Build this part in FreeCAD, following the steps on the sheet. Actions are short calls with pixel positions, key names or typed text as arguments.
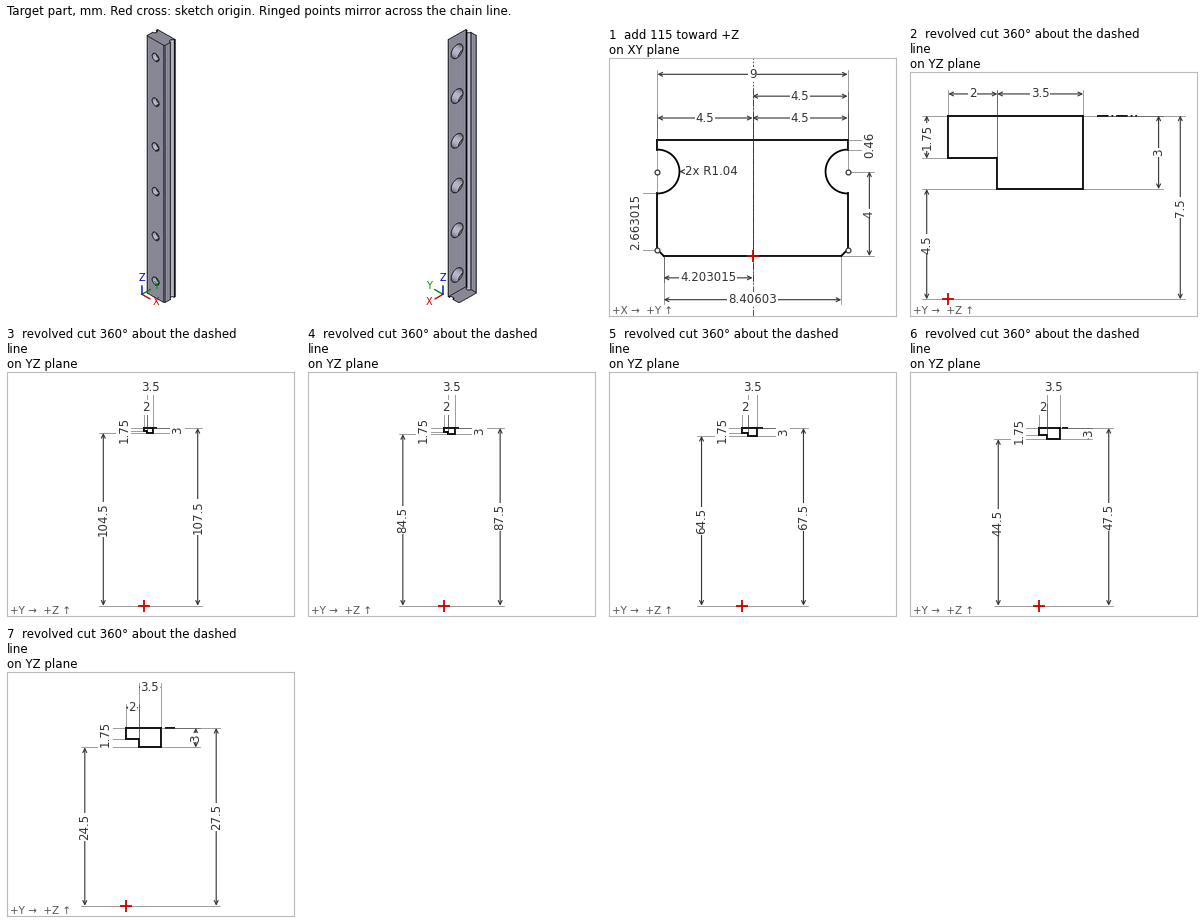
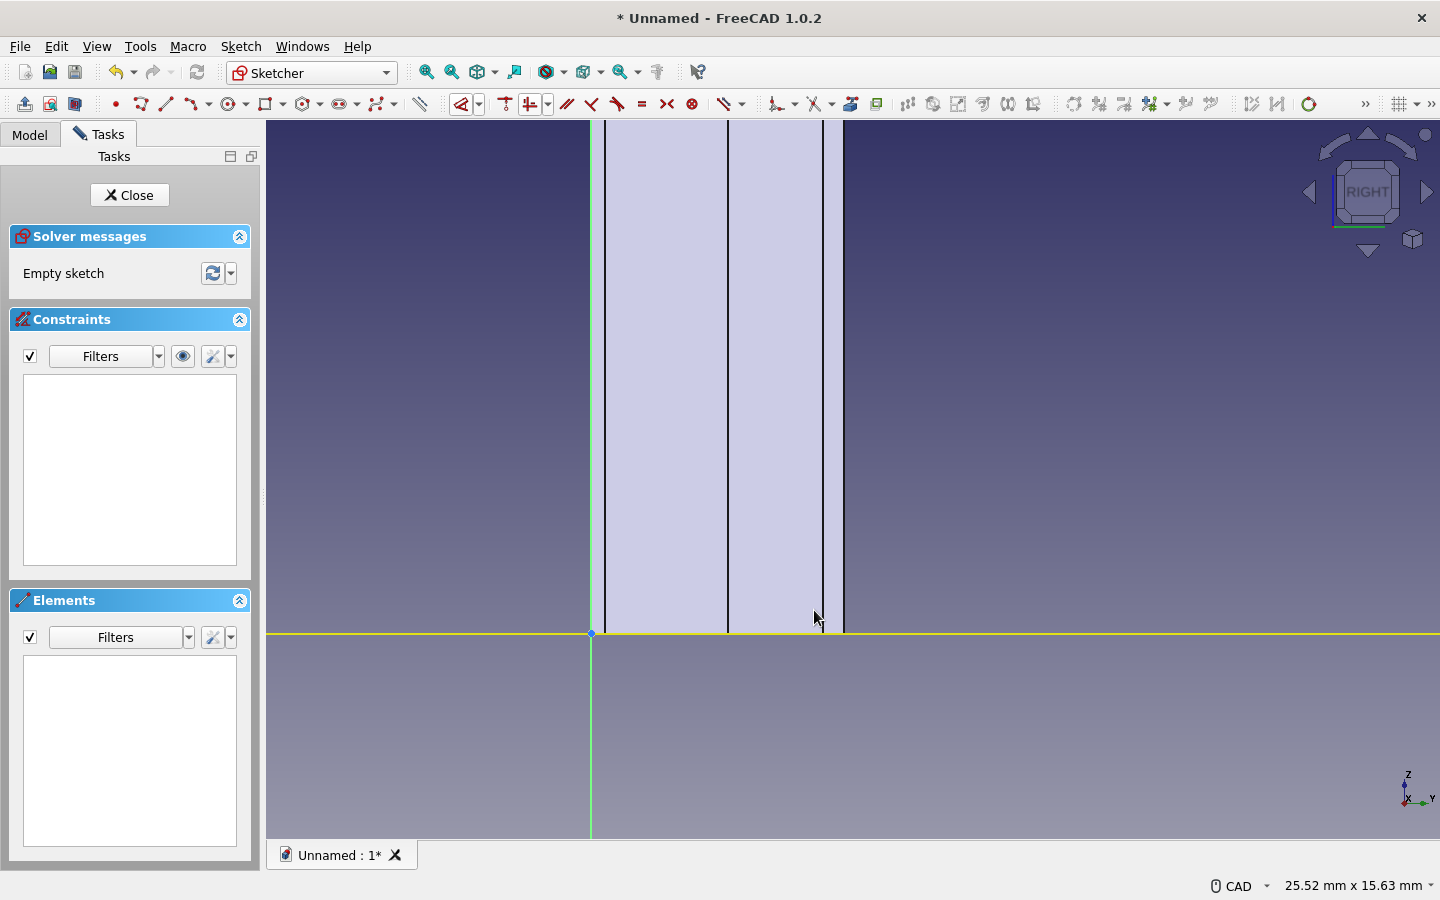
scroll(736, 424, up, 2)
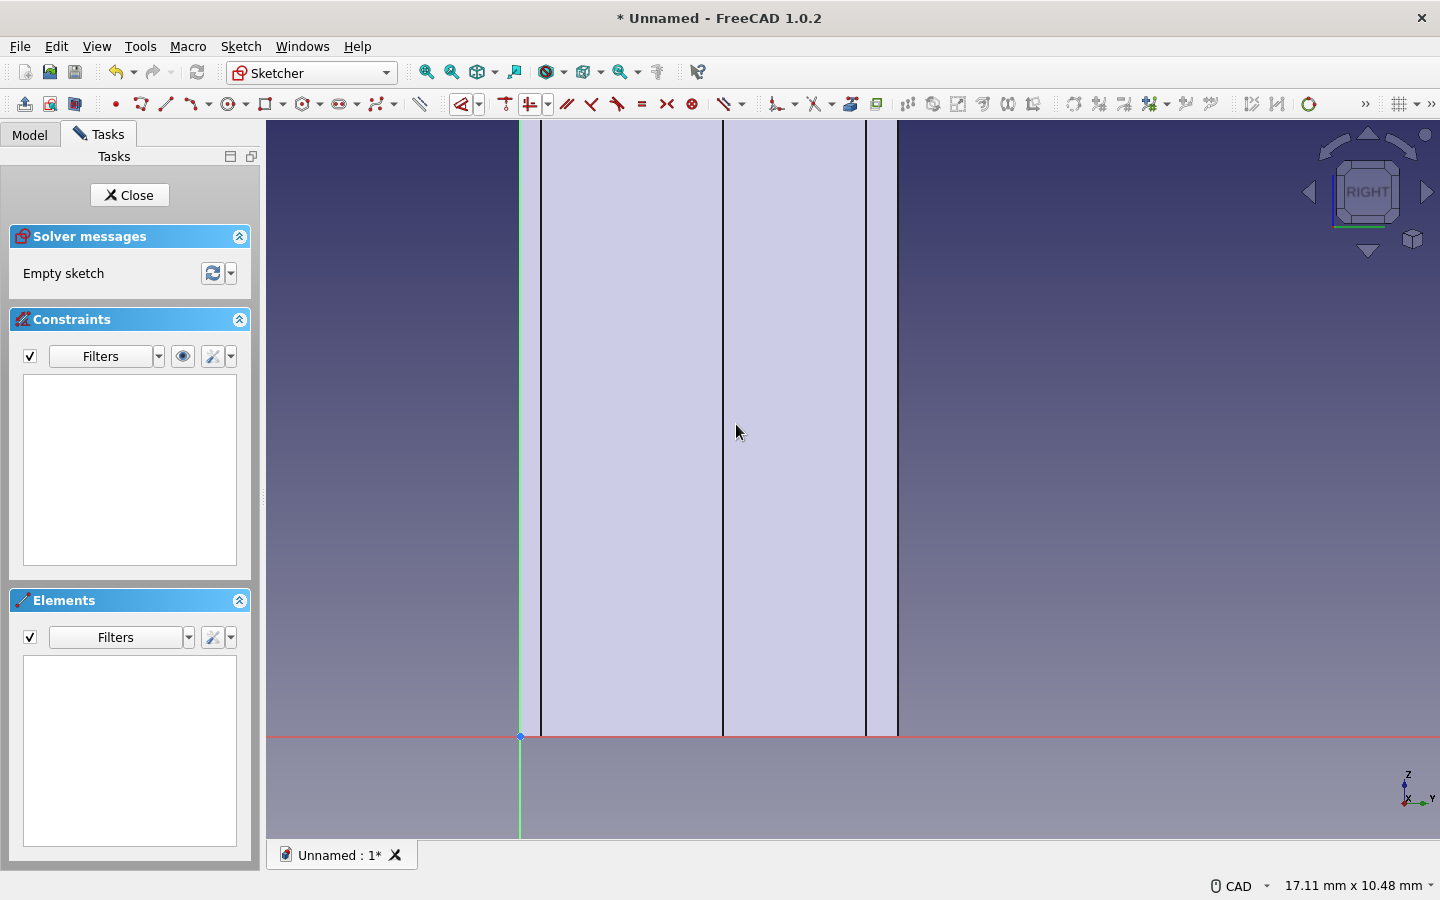
click(141, 104)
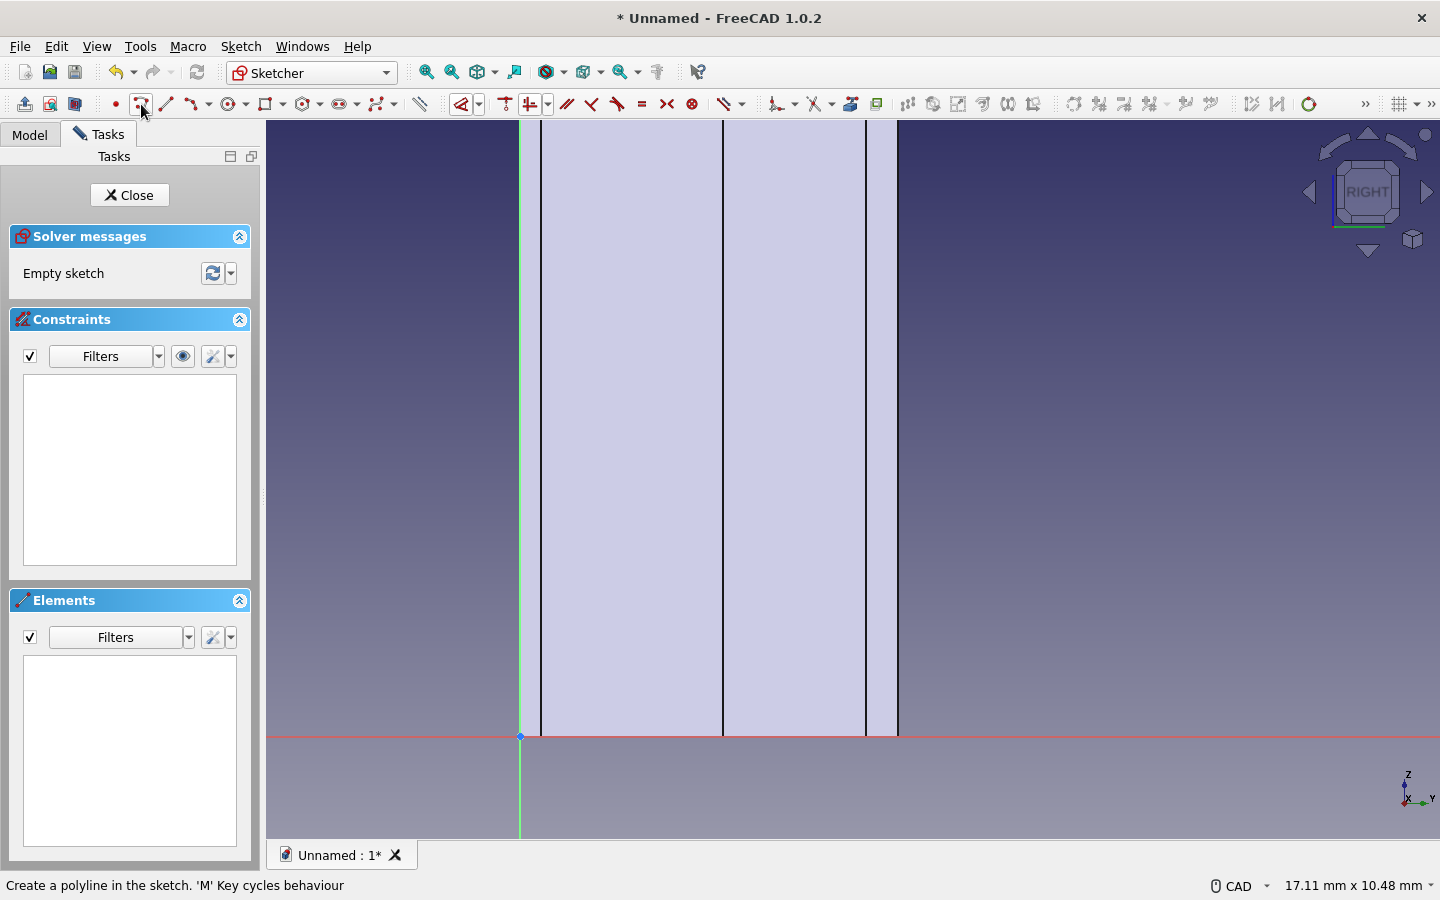
click(657, 428)
click(898, 428)
click(898, 222)
click(520, 222)
click(529, 342)
click(657, 342)
click(657, 429)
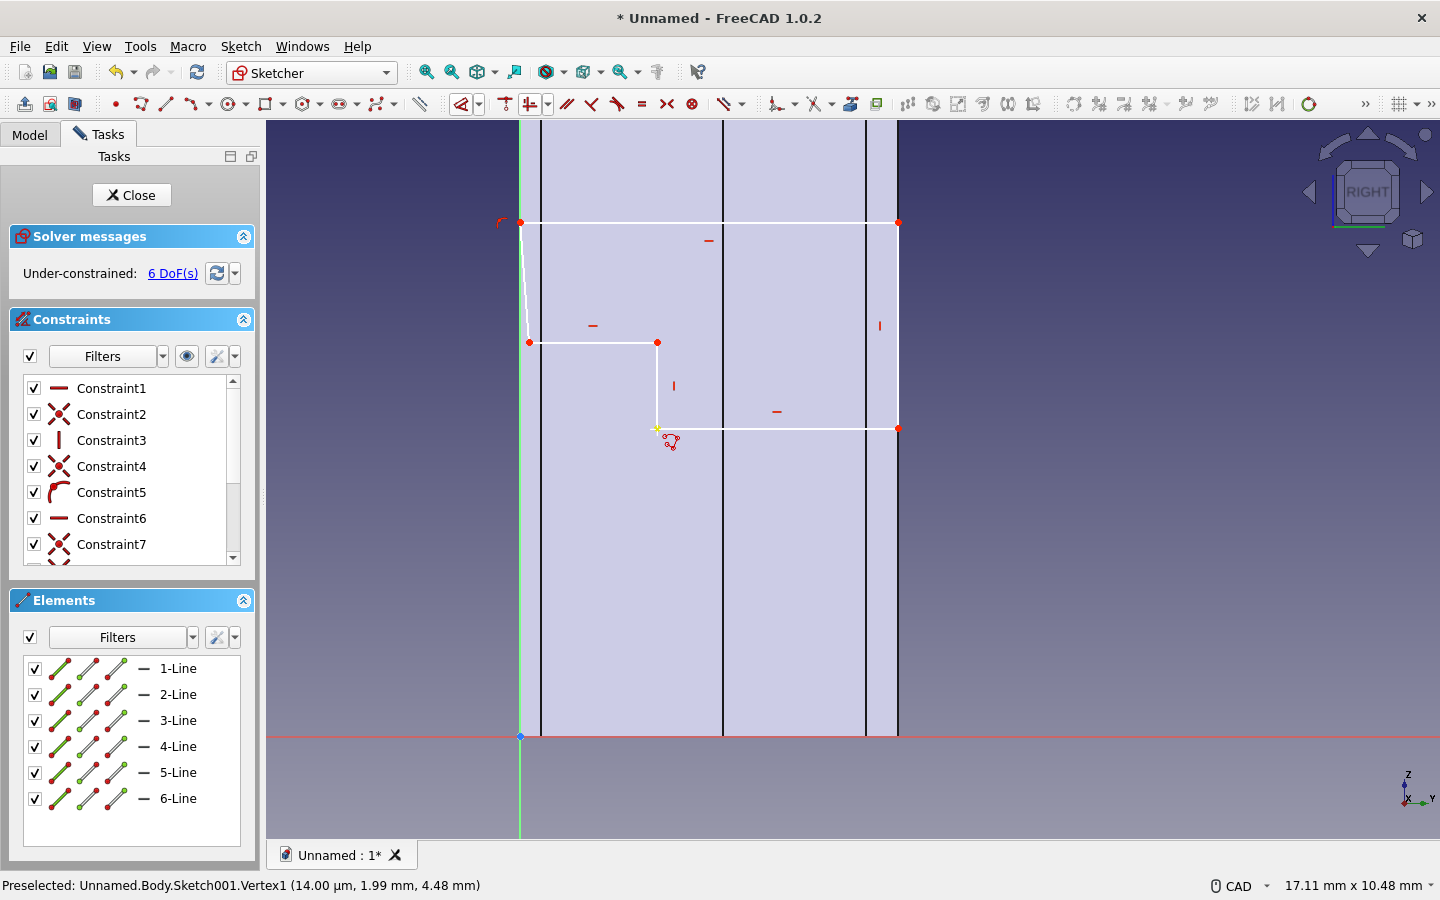
key(g)
key(l)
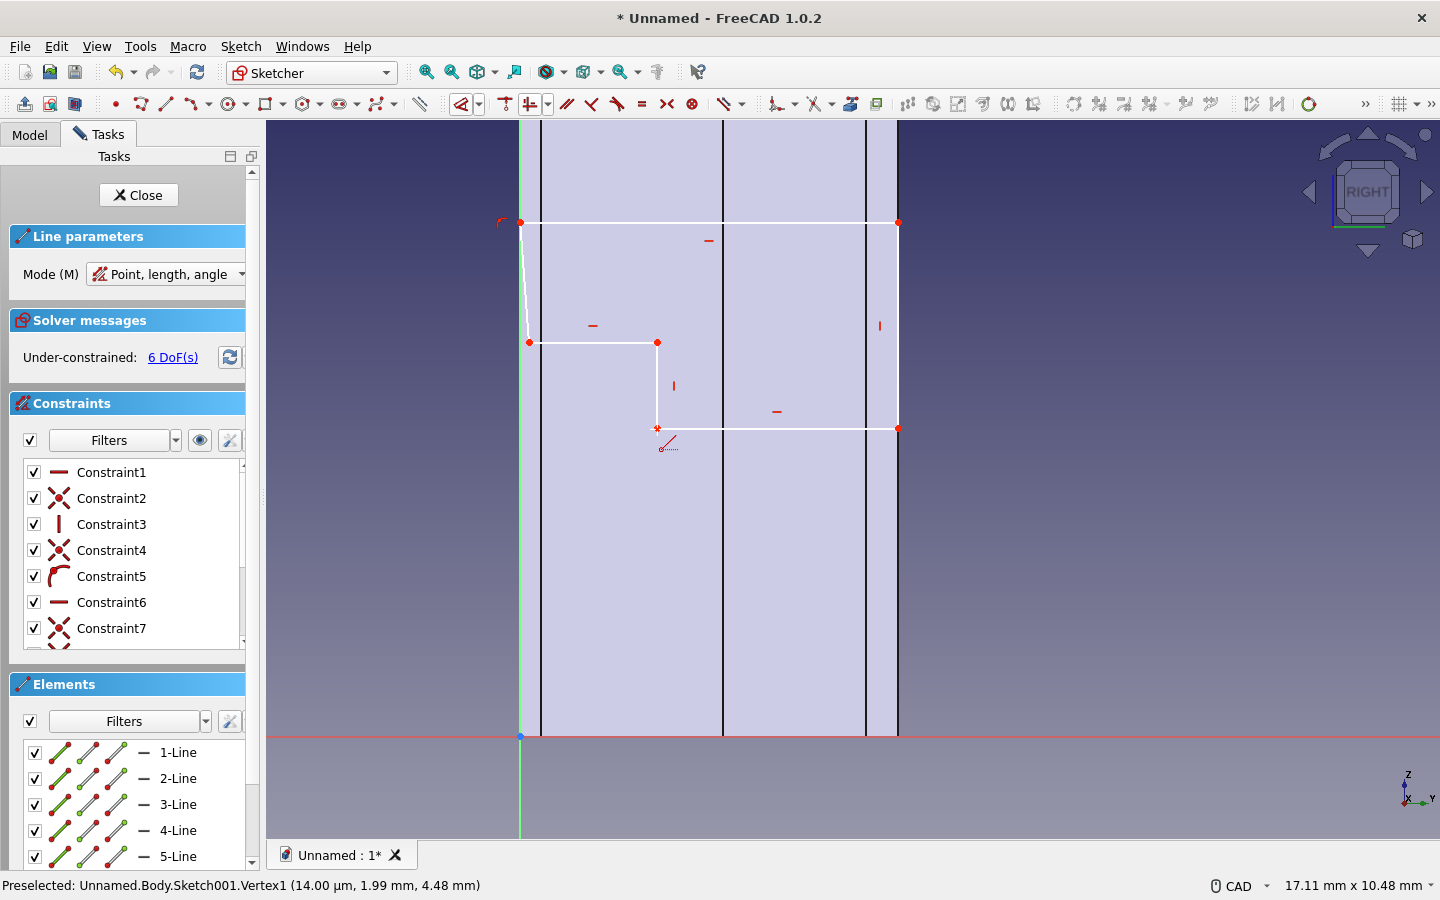
click(935, 222)
click(1049, 222)
key(Escape)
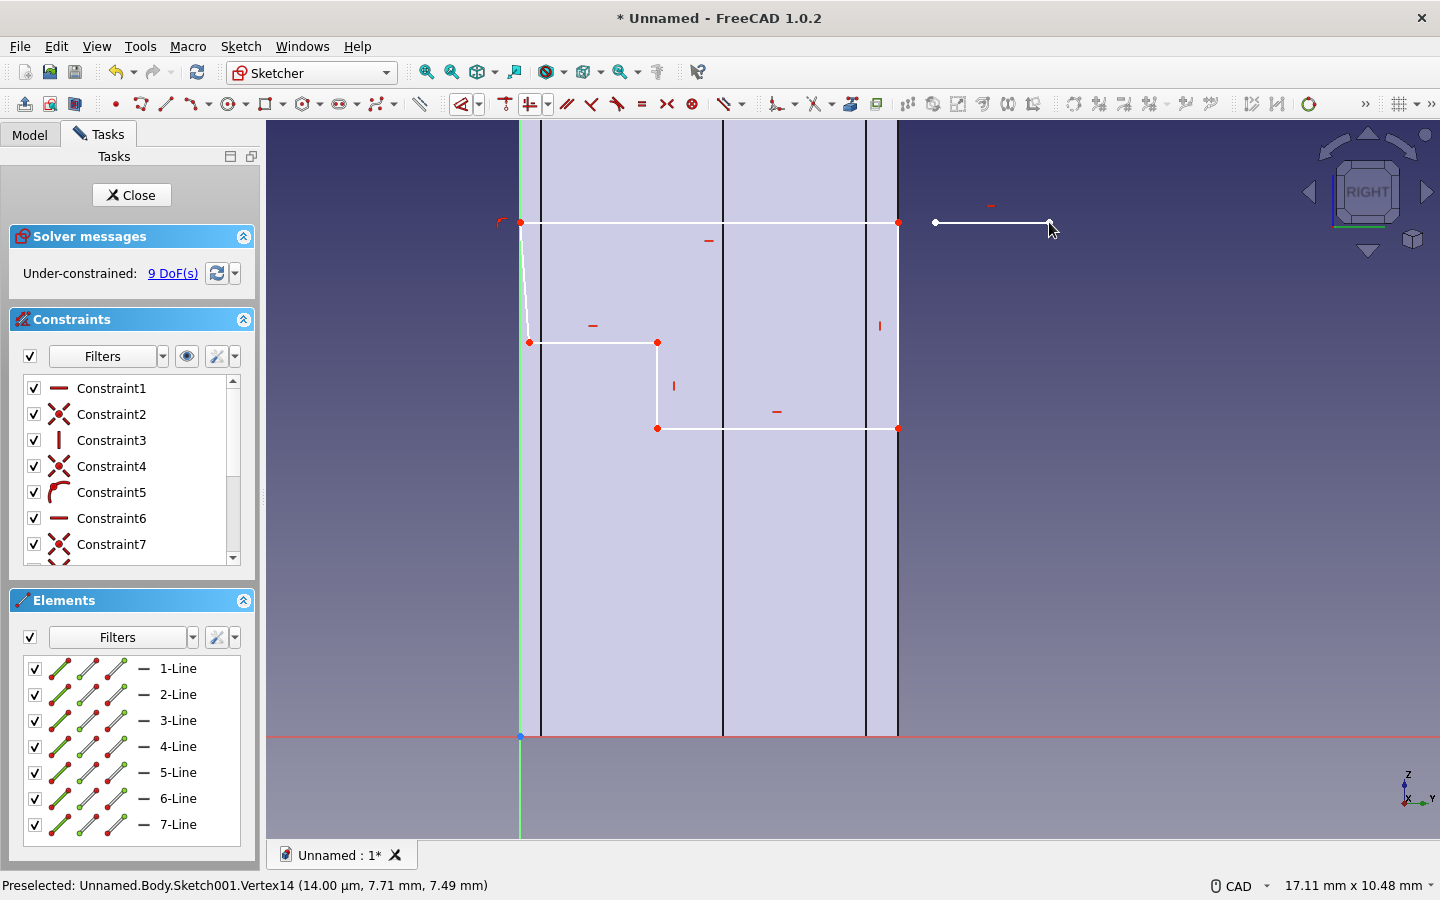
click(969, 223)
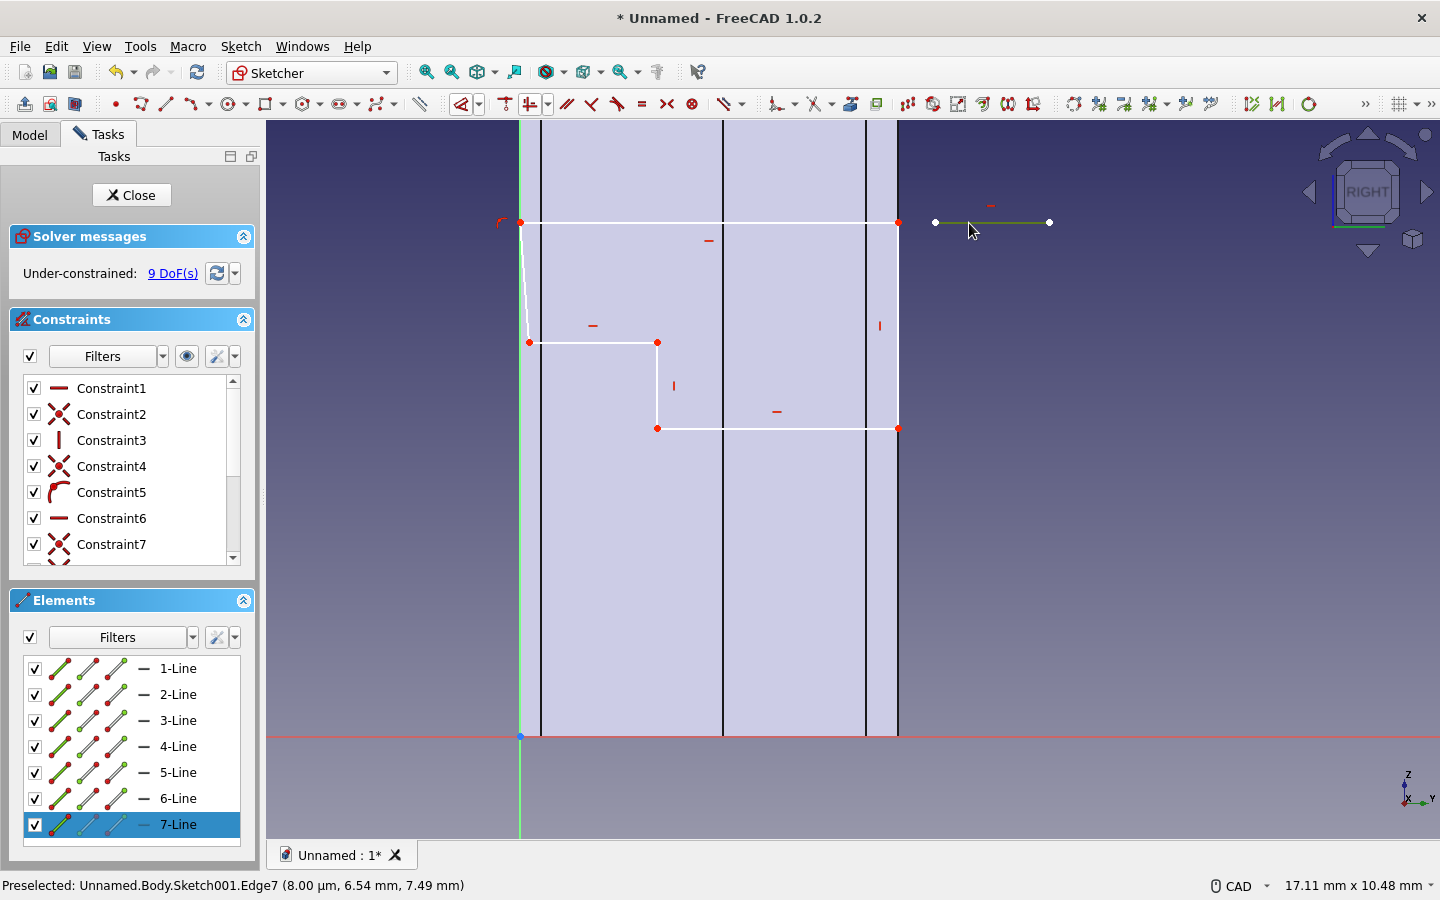
click(420, 104)